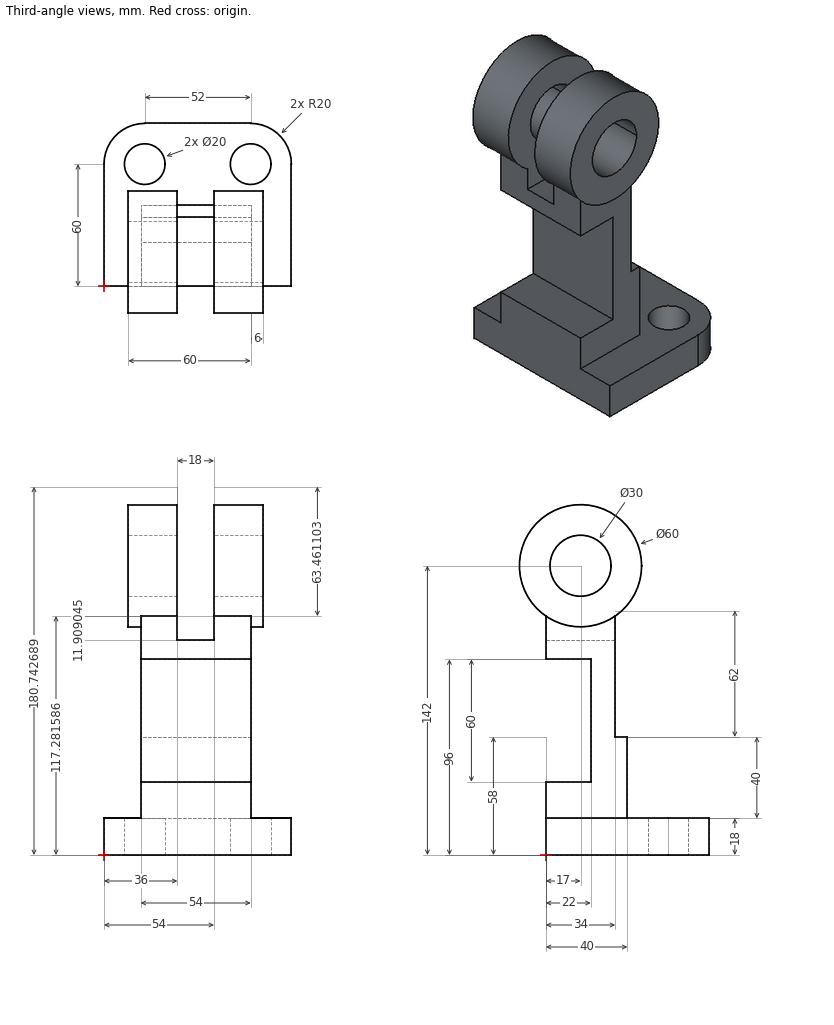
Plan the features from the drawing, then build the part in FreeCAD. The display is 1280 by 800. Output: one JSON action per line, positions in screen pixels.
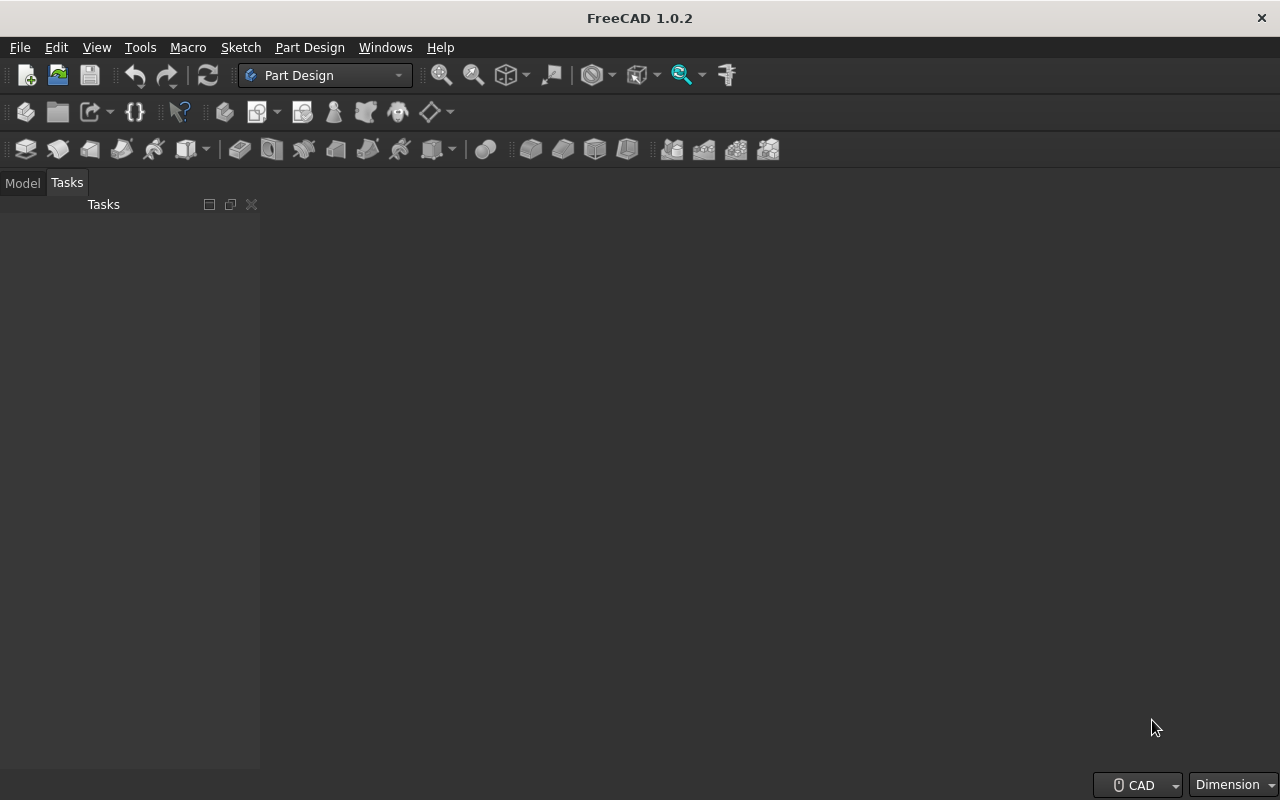
{"action": "left_click", "coordinate": [26, 76]}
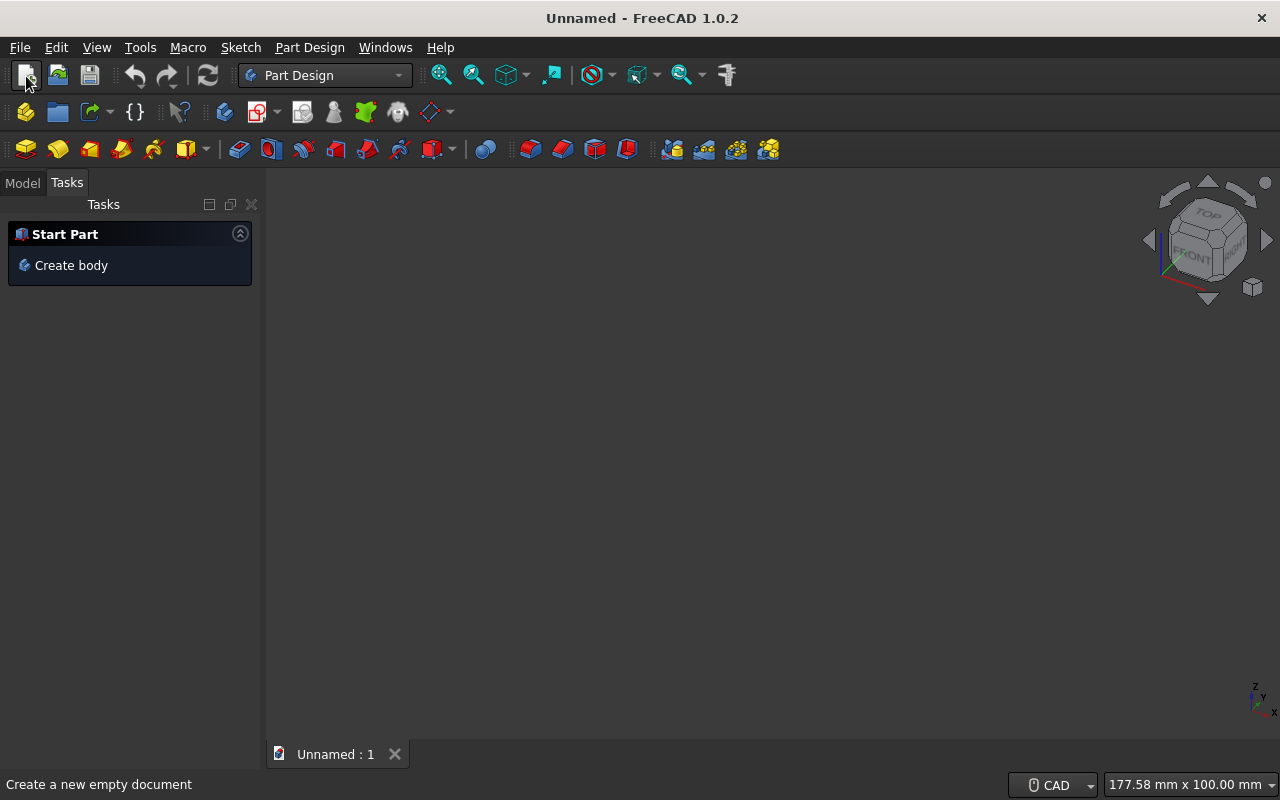
{"action": "left_click", "coordinate": [258, 112]}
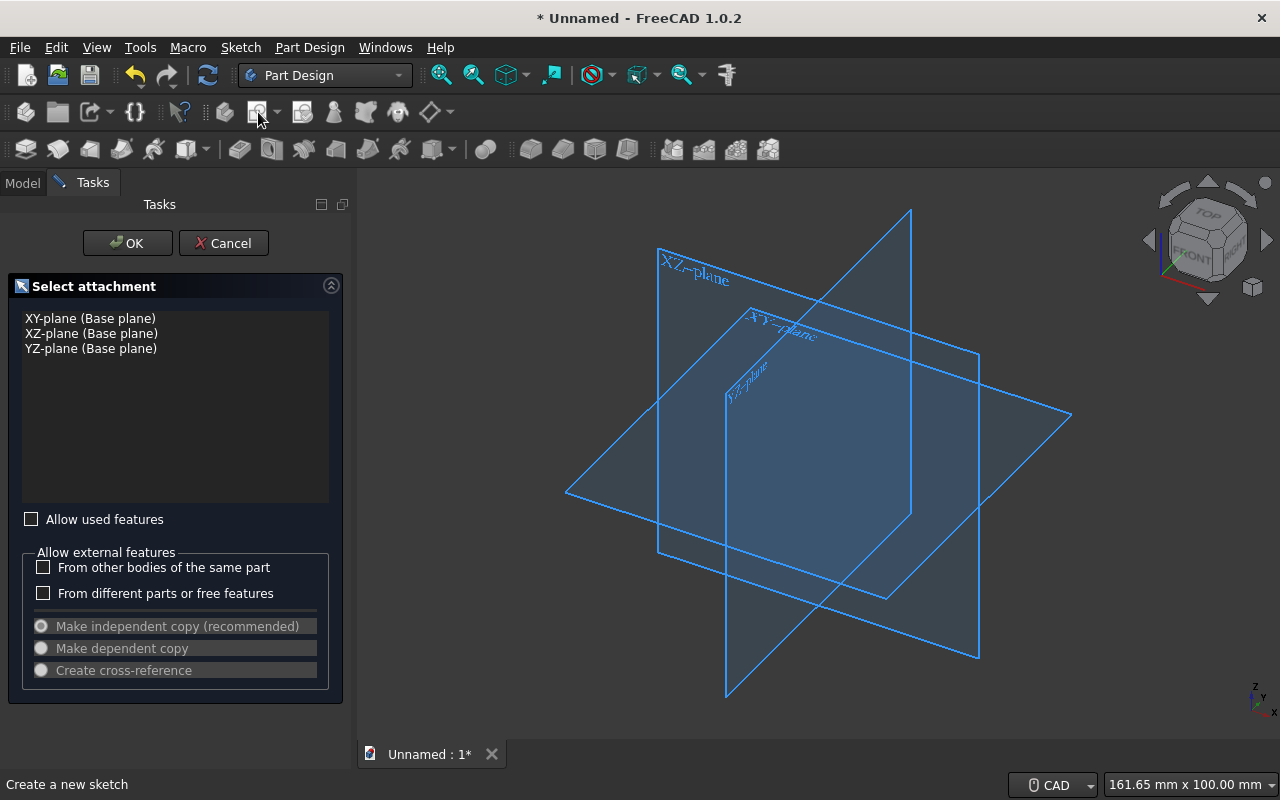
{"action": "left_click", "coordinate": [82, 318]}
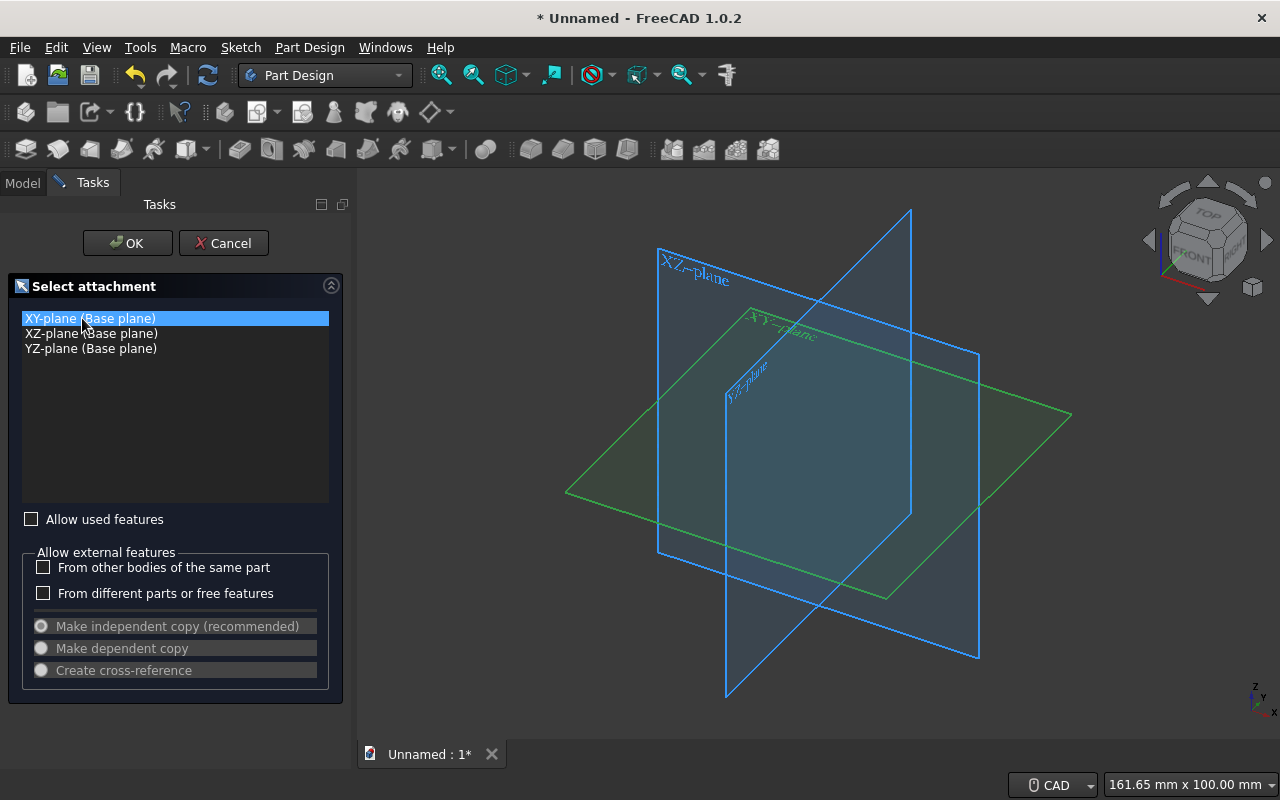
{"action": "left_click", "coordinate": [128, 243]}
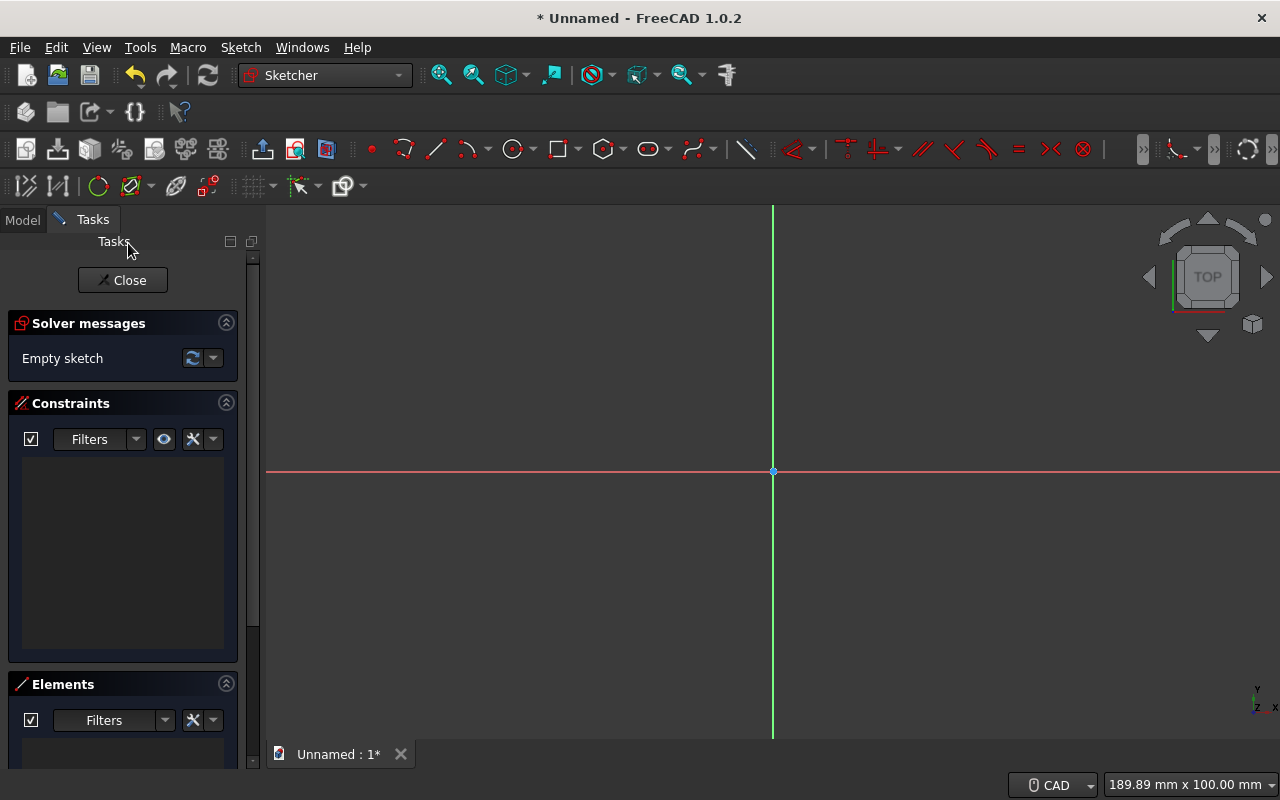
{"action": "scroll", "coordinate": [294, 711], "scroll_direction": "down", "scroll_amount": 2}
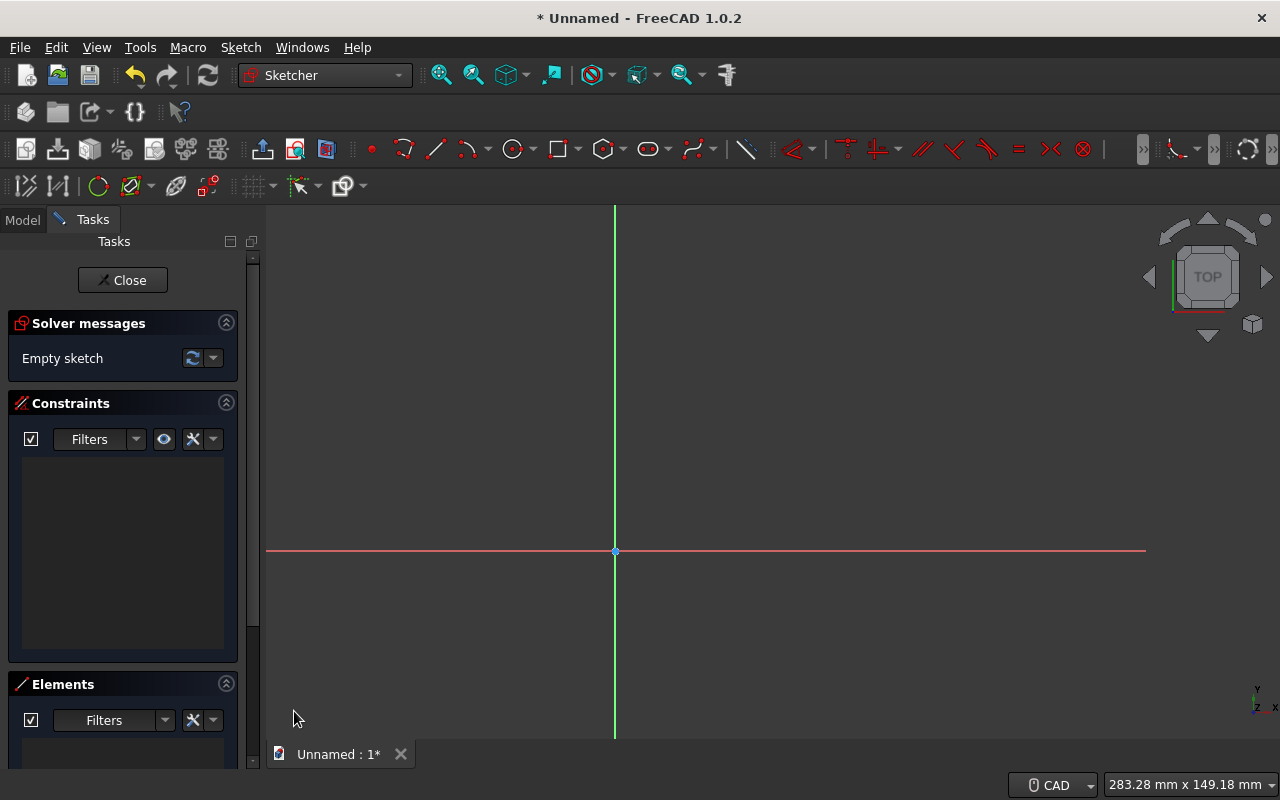
{"action": "left_click", "coordinate": [436, 150]}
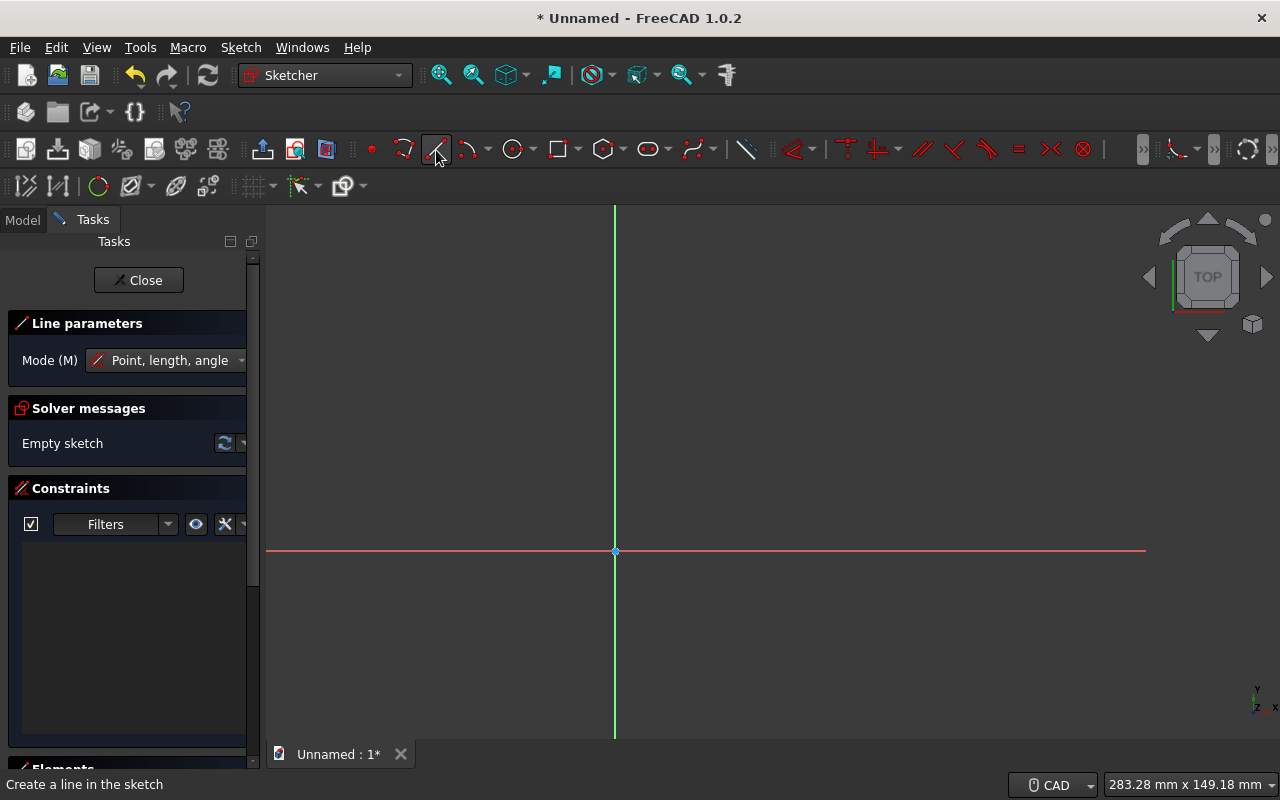
{"action": "left_click", "coordinate": [873, 265]}
{"action": "left_click", "coordinate": [687, 265]}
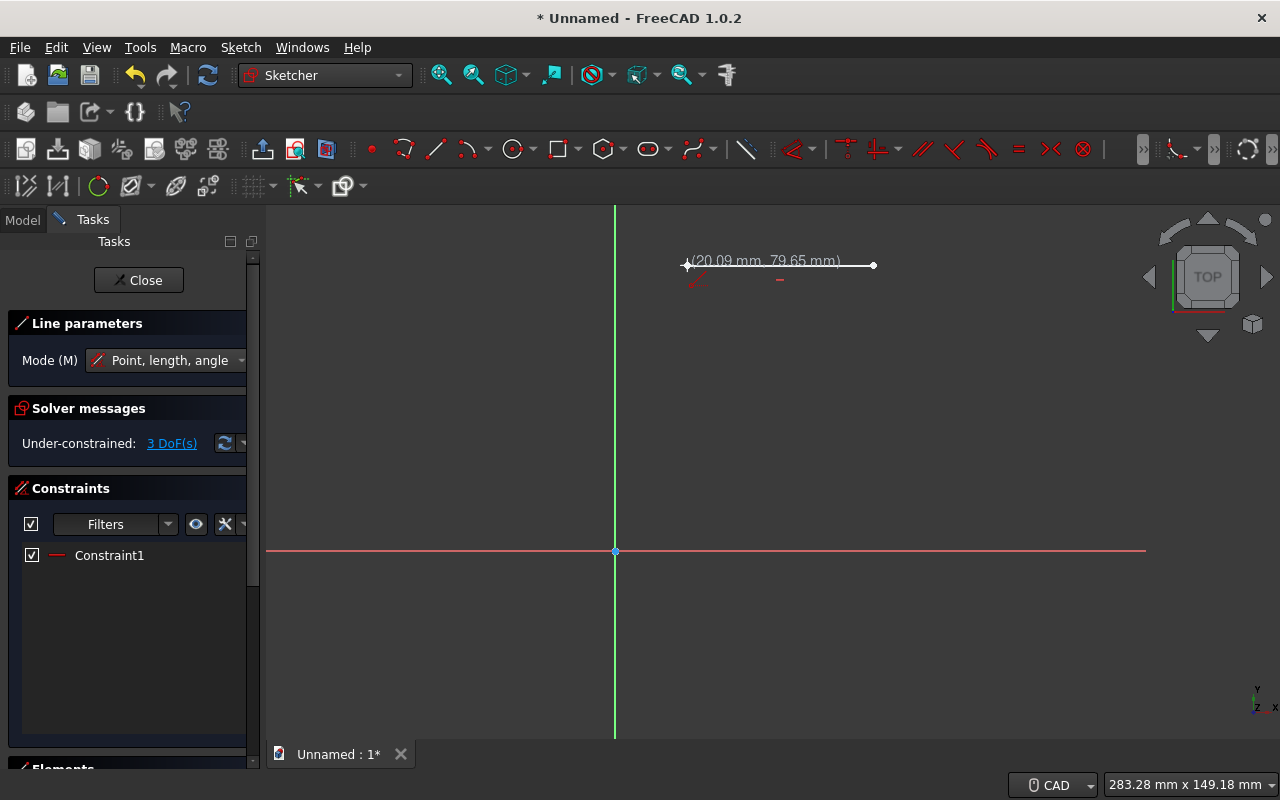
{"action": "left_click", "coordinate": [404, 150]}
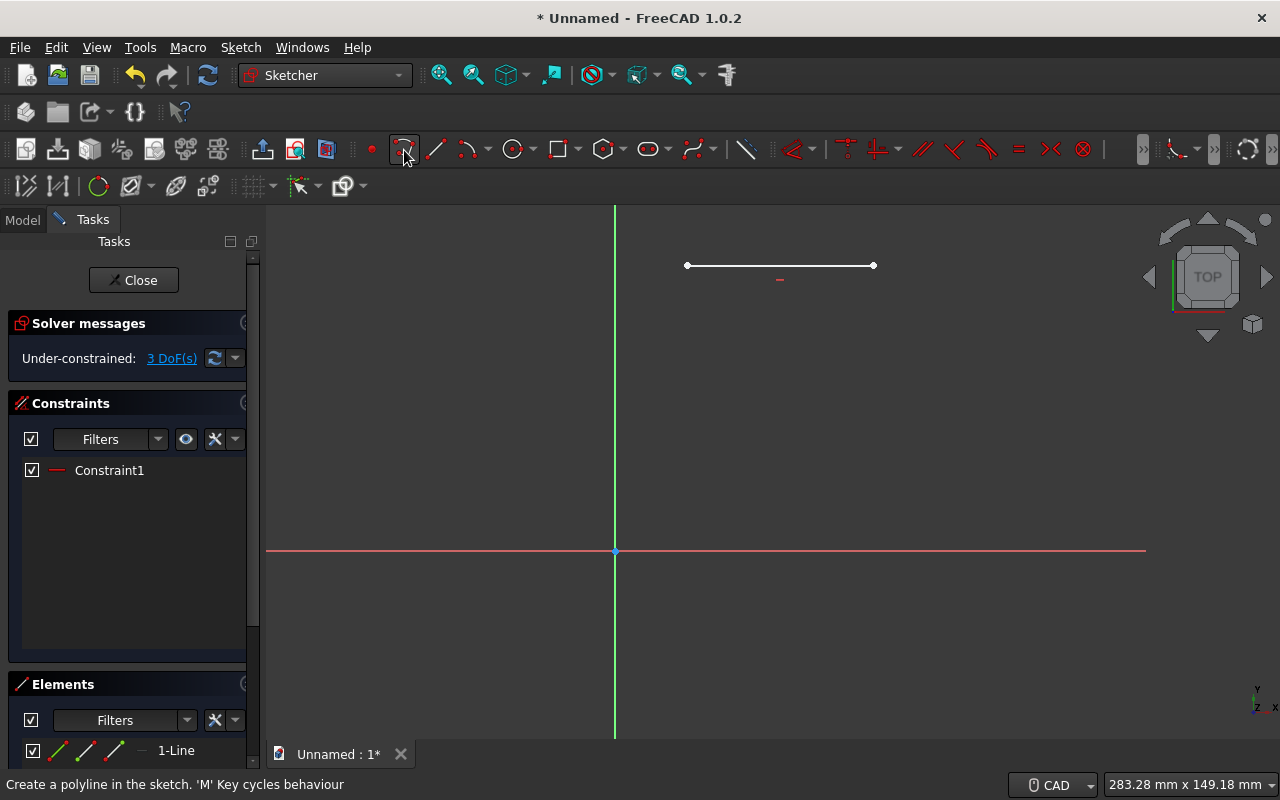
{"action": "left_click", "coordinate": [615, 336]}
{"action": "left_click", "coordinate": [615, 551]}
{"action": "left_click", "coordinate": [944, 542]}
{"action": "left_click", "coordinate": [944, 336]}
{"action": "right_click", "coordinate": [944, 336]}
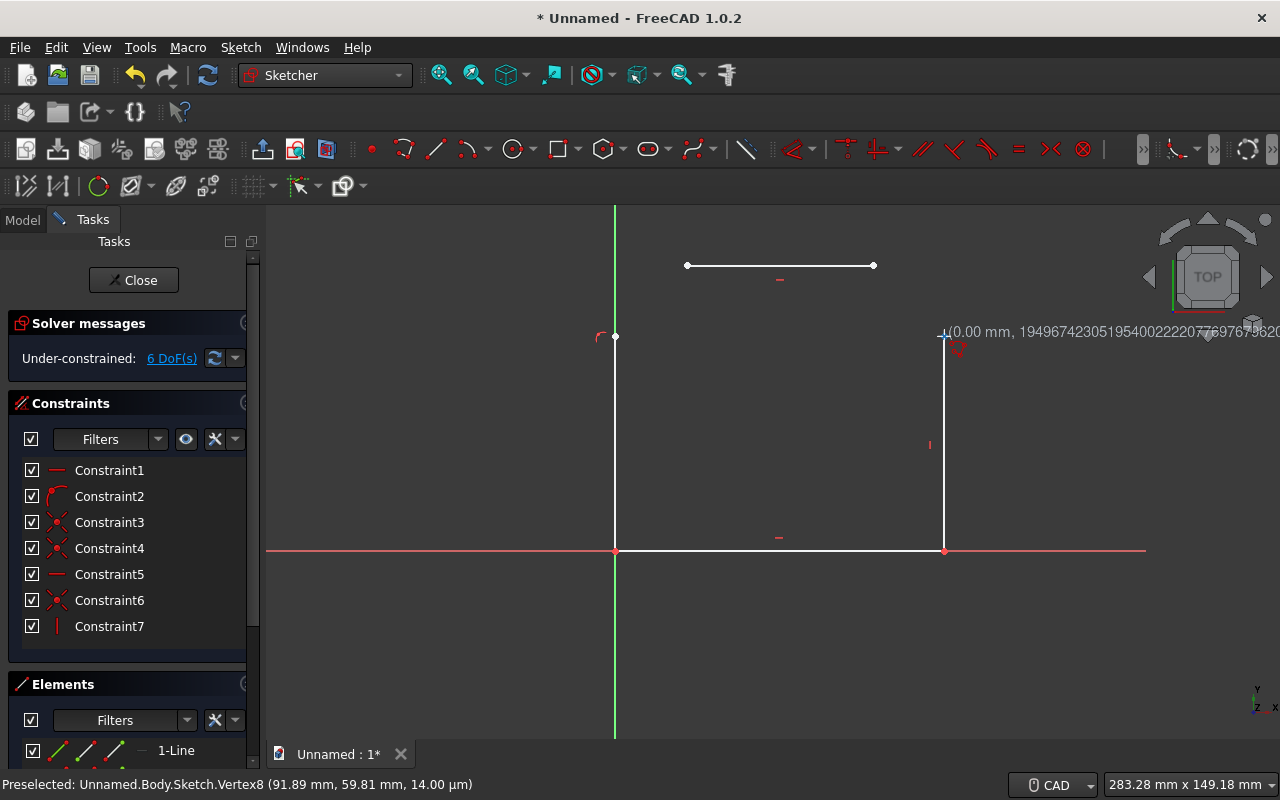
{"action": "left_click", "coordinate": [490, 150]}